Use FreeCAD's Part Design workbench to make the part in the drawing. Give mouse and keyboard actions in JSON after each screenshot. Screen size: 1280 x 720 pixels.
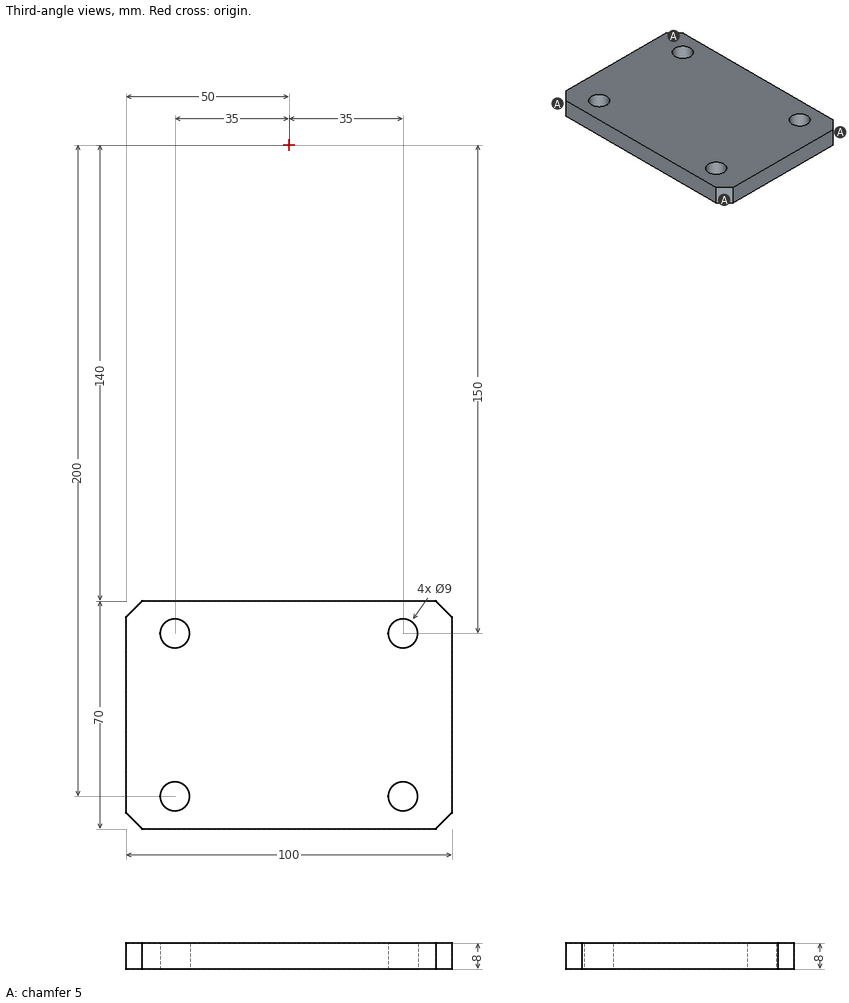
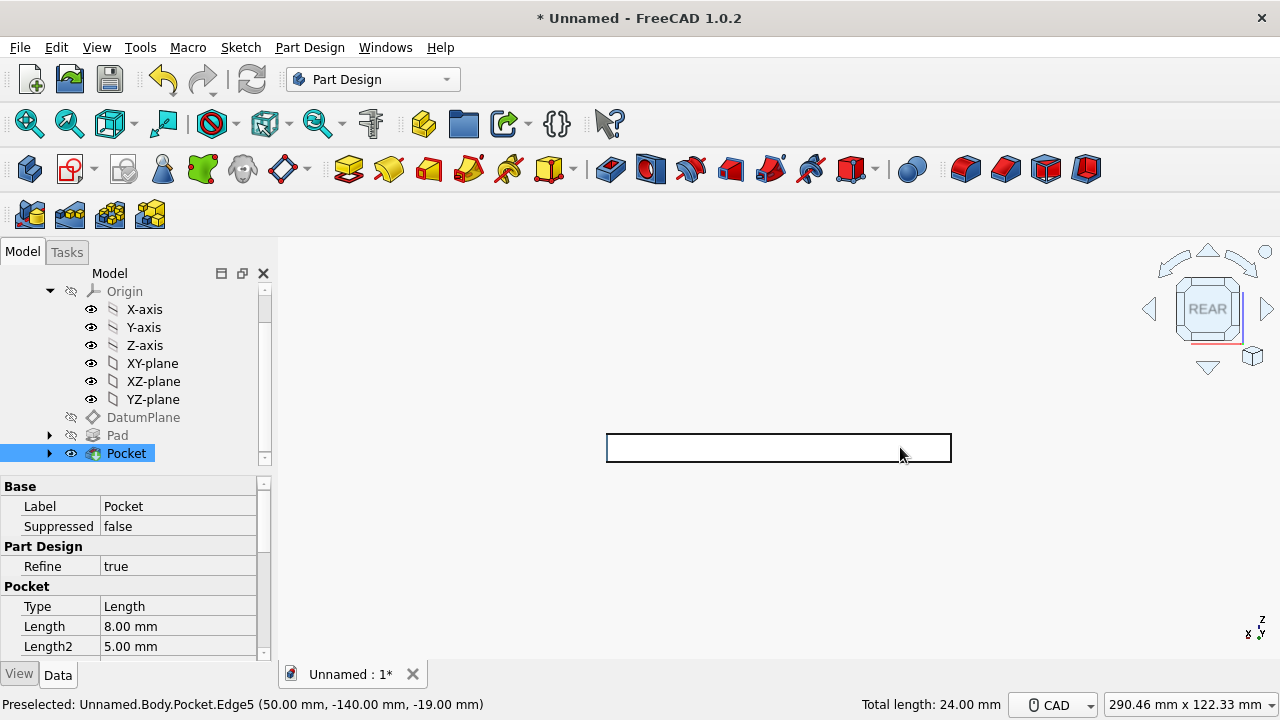
{"action": "left_click", "coordinate": [30, 124]}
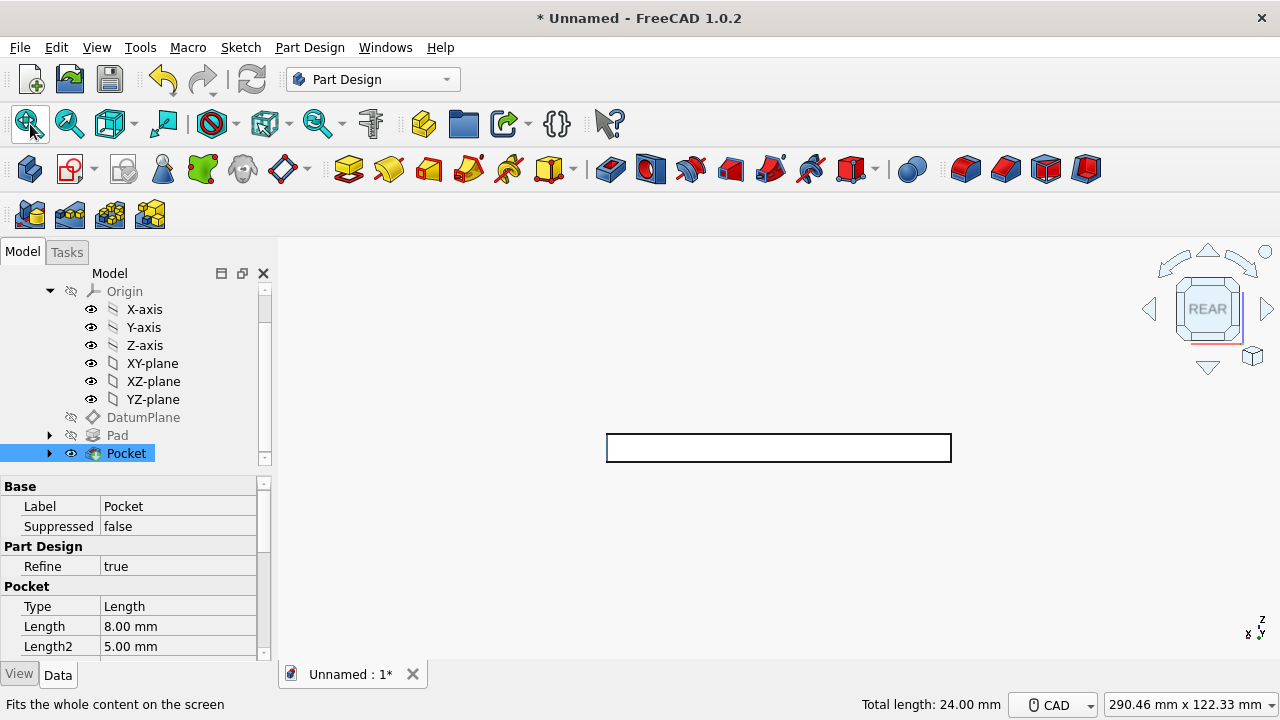
{"action": "left_click", "coordinate": [951, 447], "text": "ctrl"}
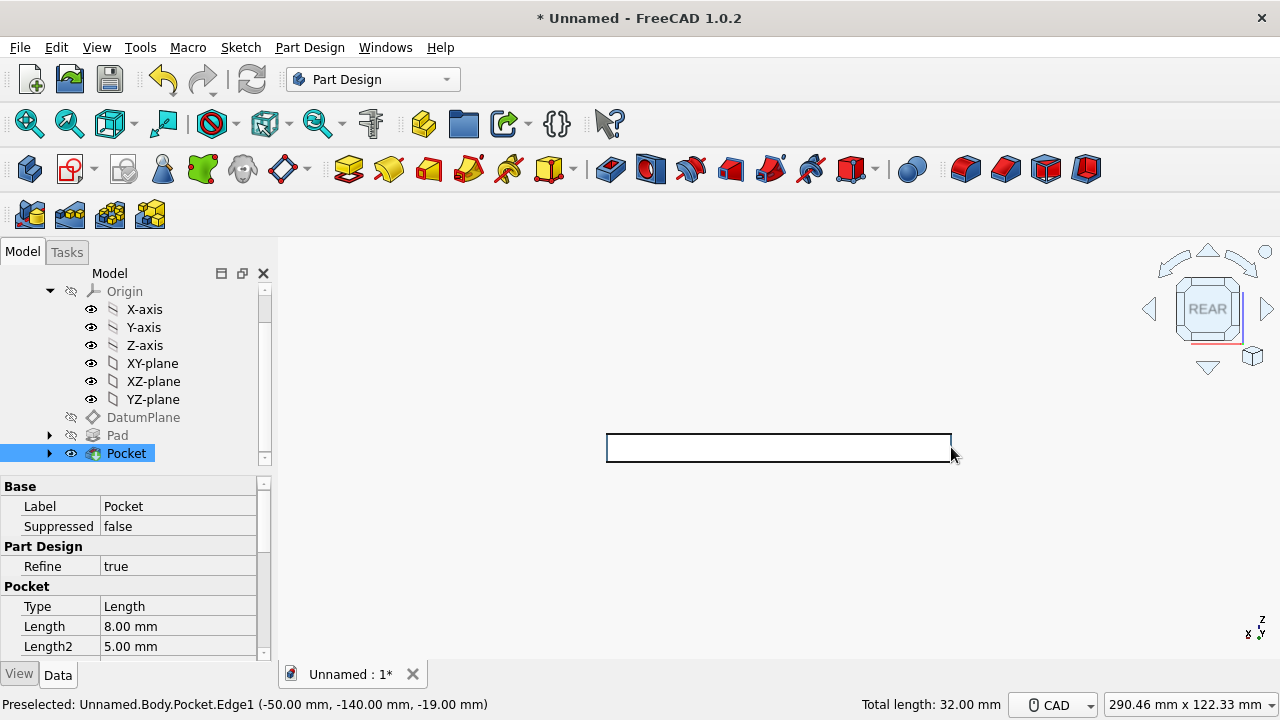
{"action": "left_click", "coordinate": [1006, 170]}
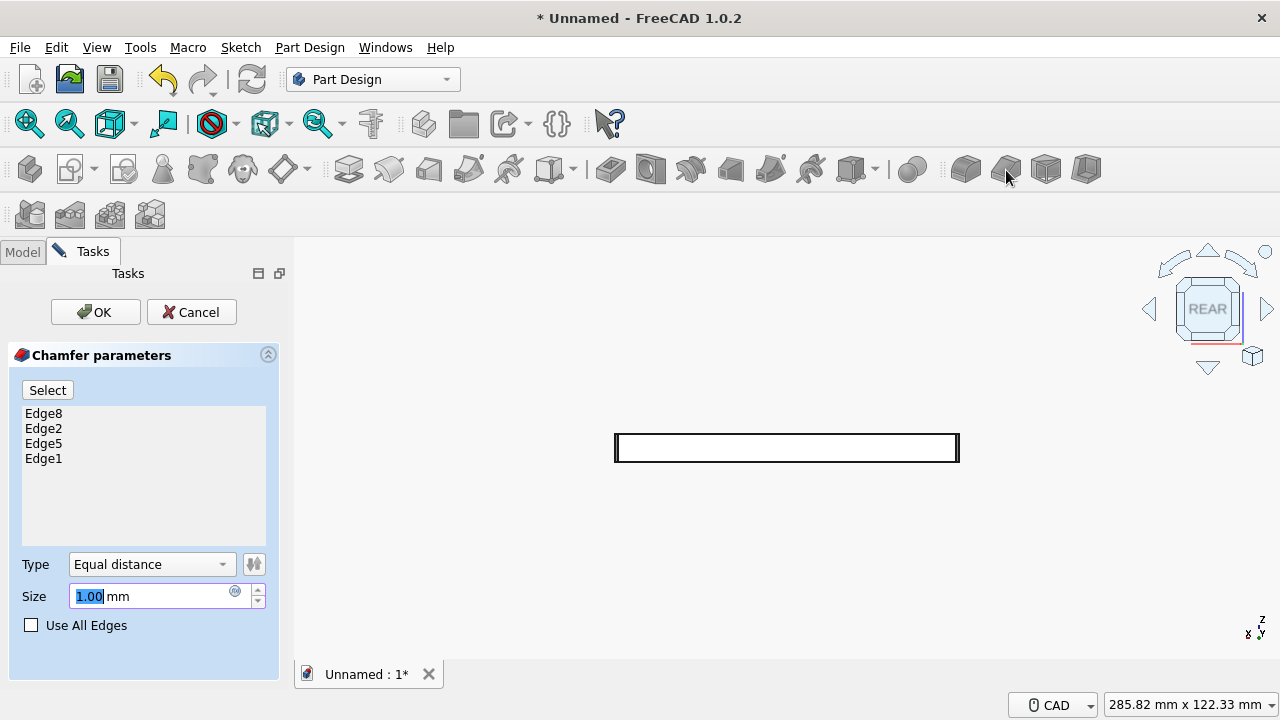
{"action": "type", "text": "5"}
{"action": "key", "text": "Tab"}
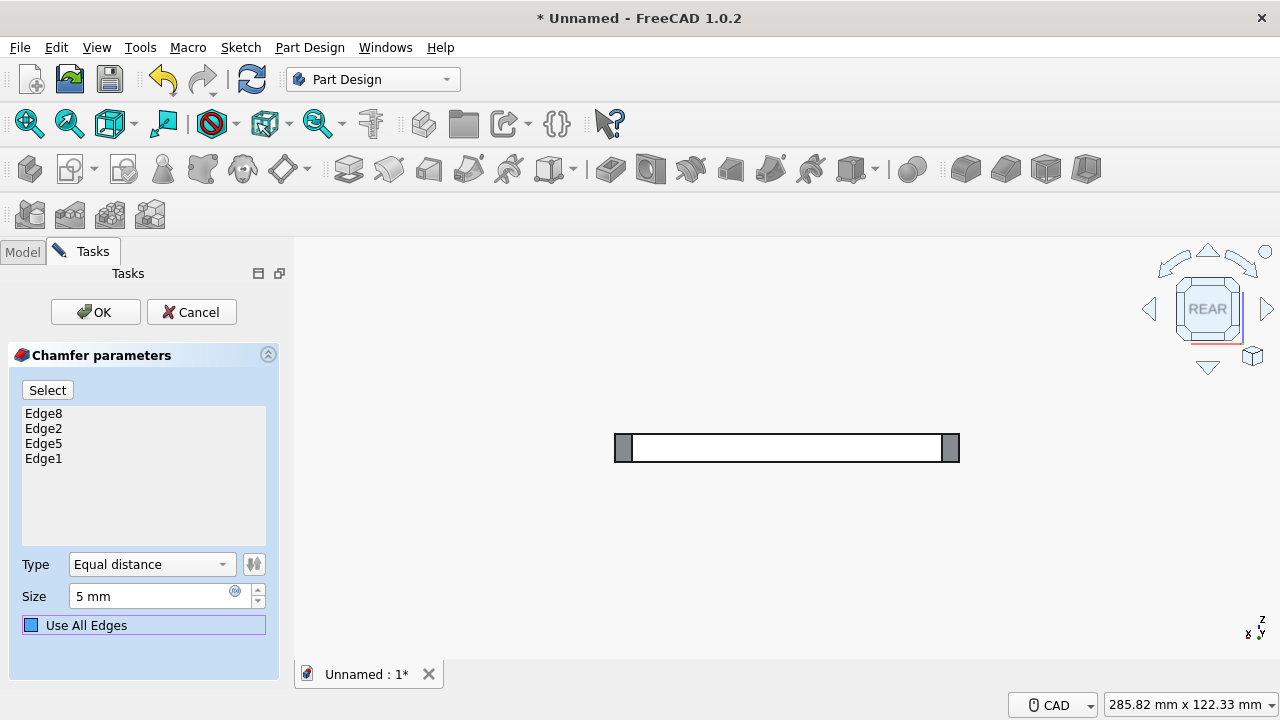
{"action": "left_click", "coordinate": [96, 312]}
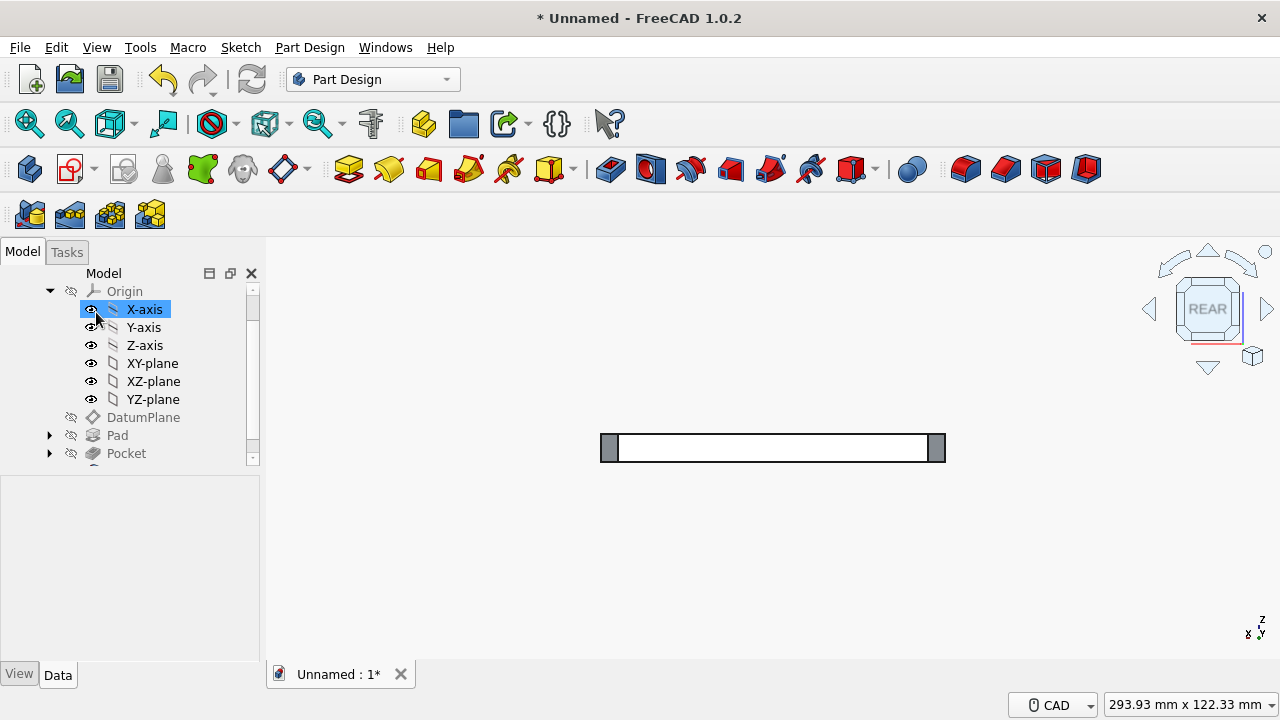
{"action": "key", "text": "0"}